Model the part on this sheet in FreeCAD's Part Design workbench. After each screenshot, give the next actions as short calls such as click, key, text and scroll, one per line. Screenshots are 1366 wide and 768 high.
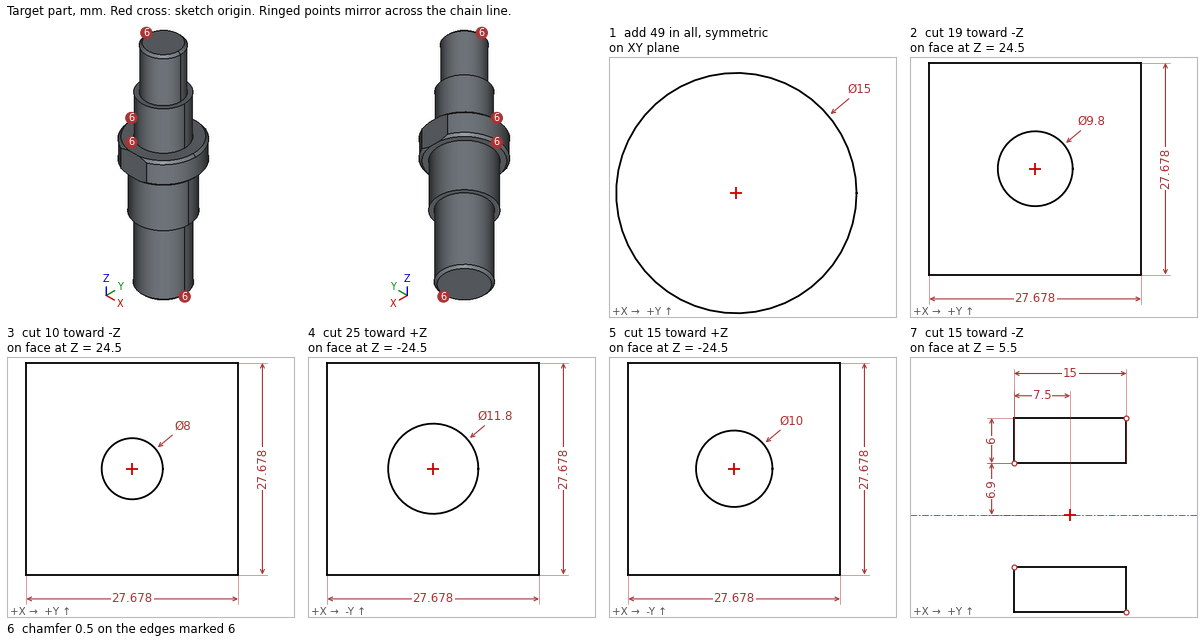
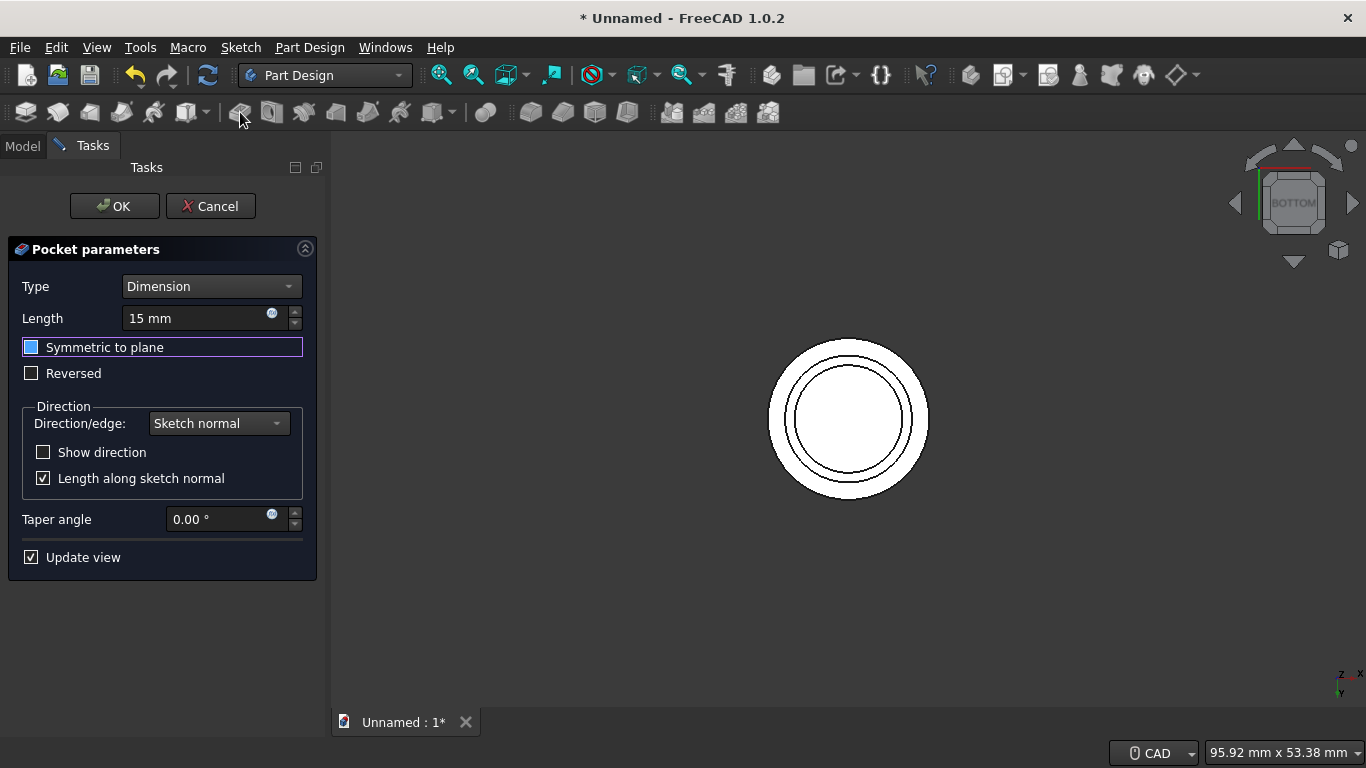
click(115, 206)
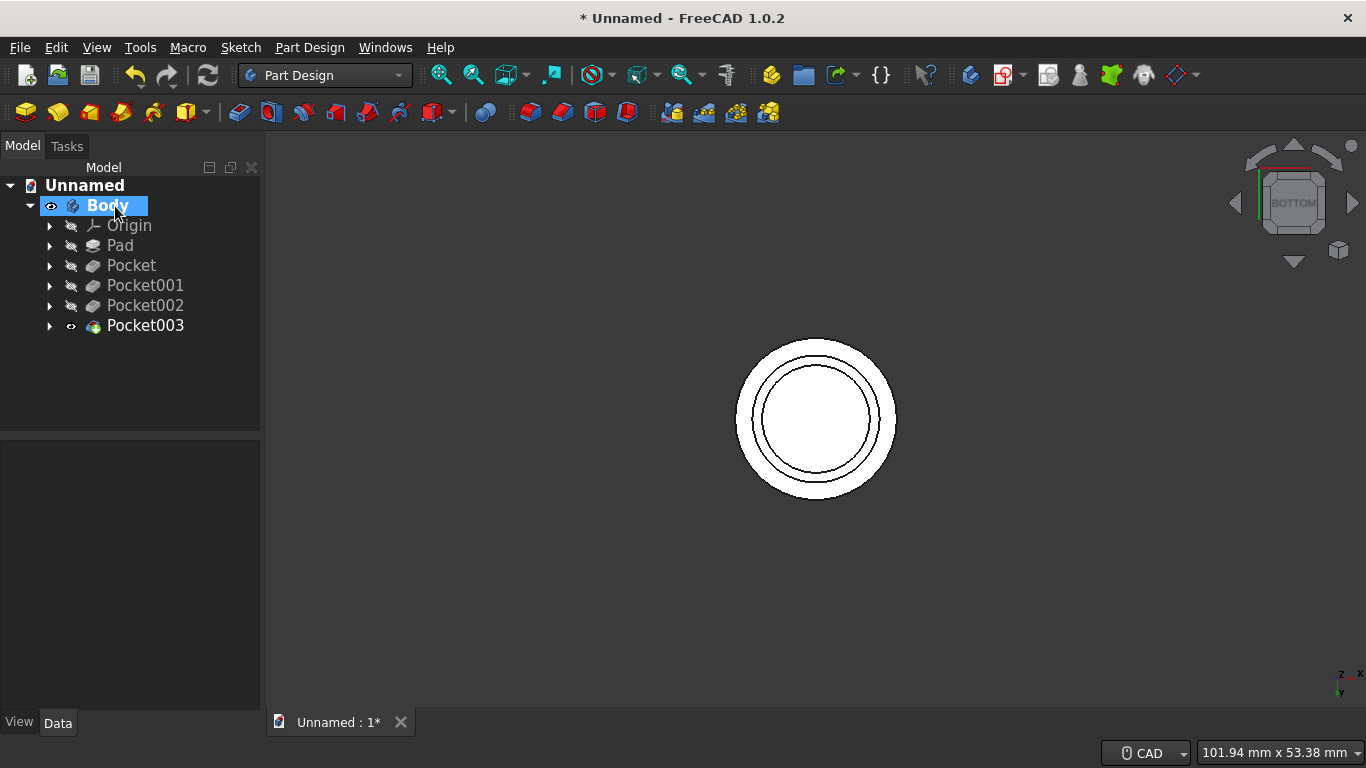
click(442, 76)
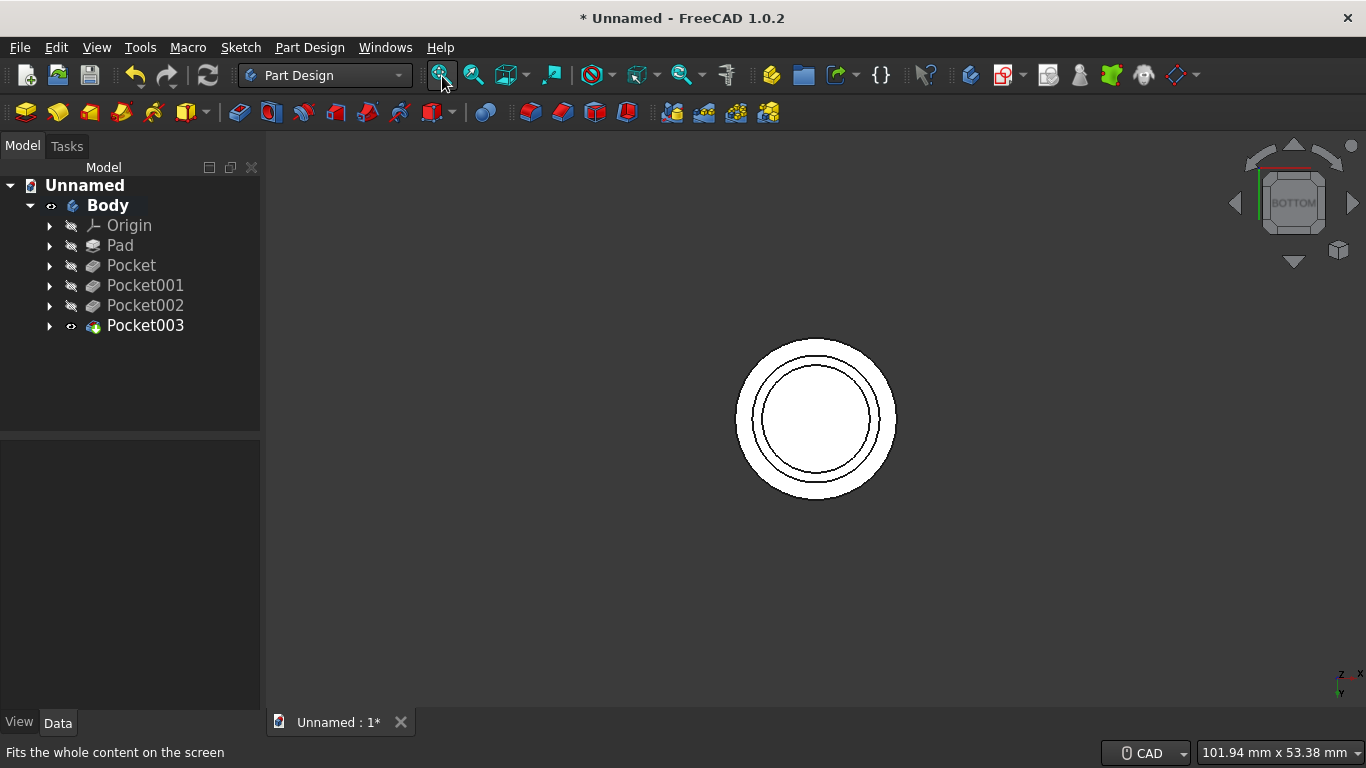
click(735, 418)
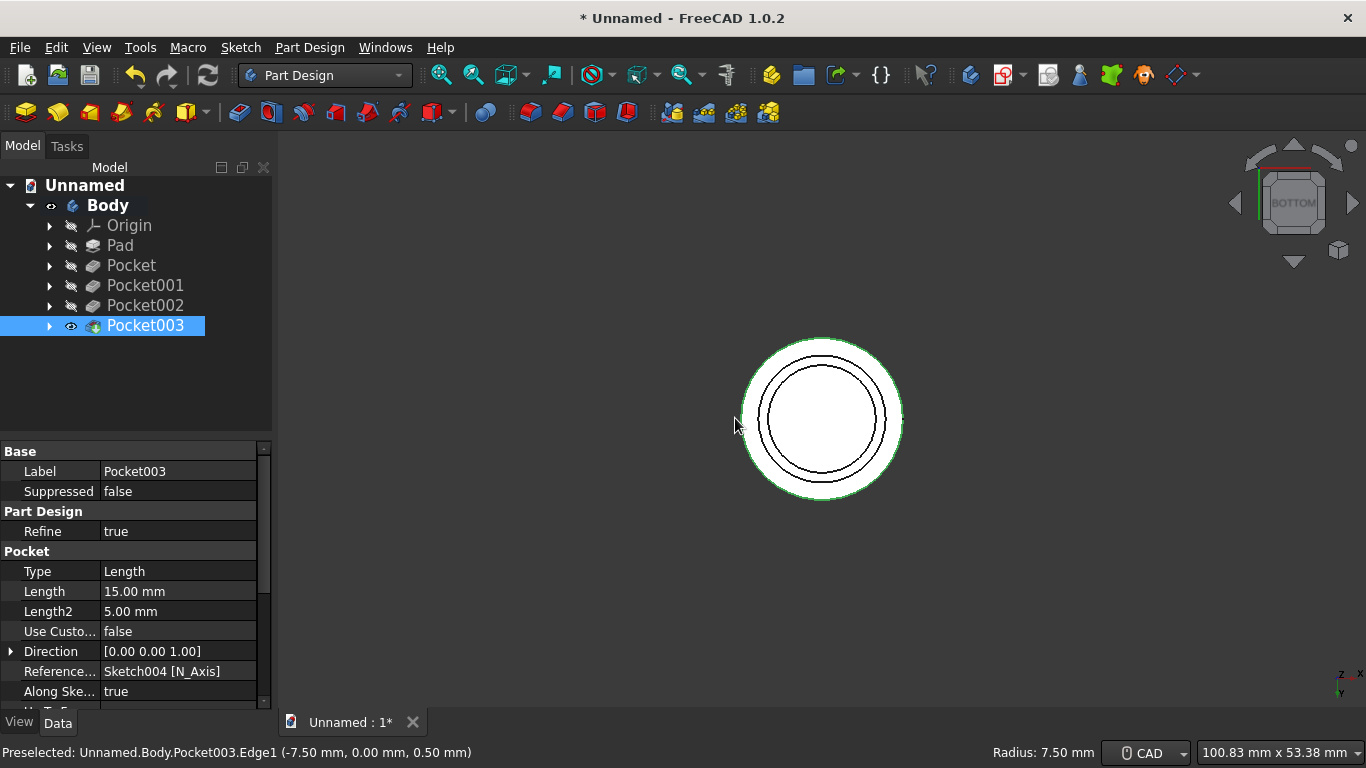
click(768, 418, ctrl)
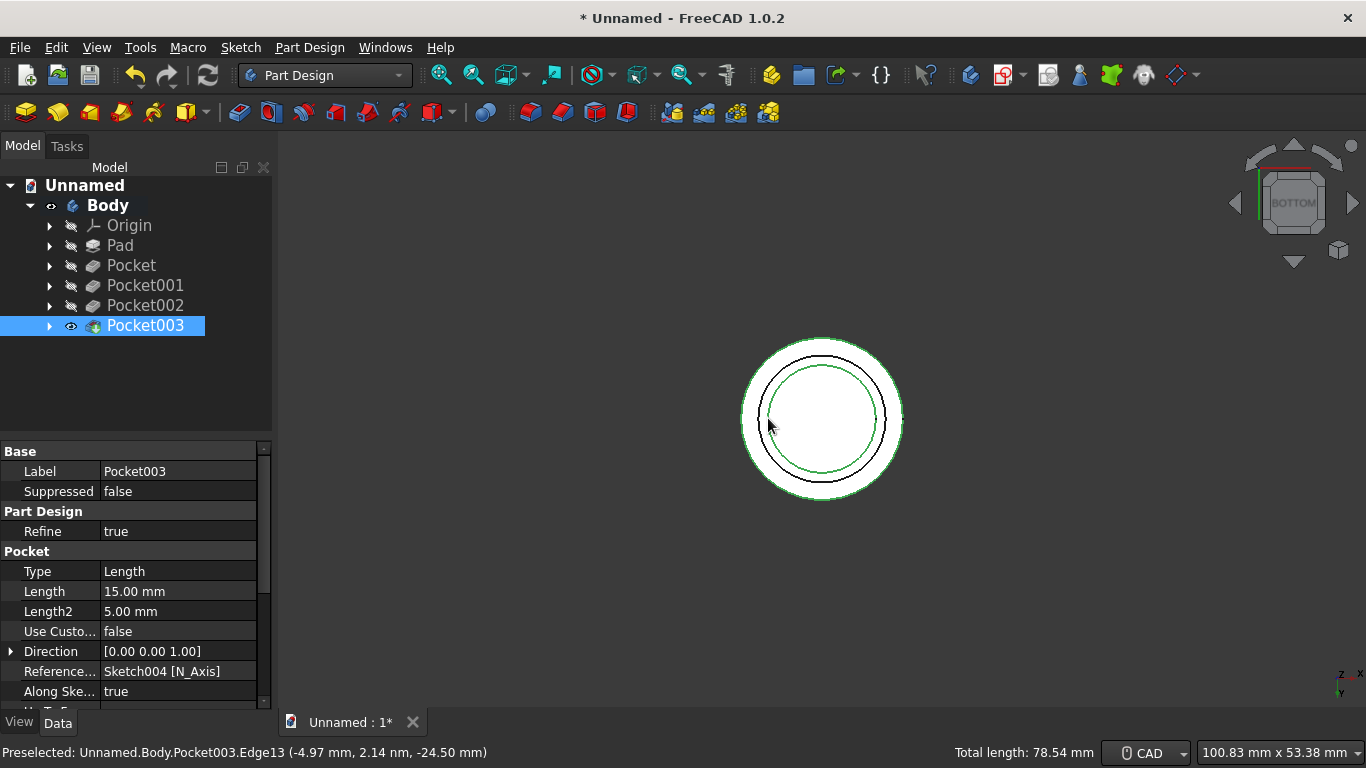
key(0)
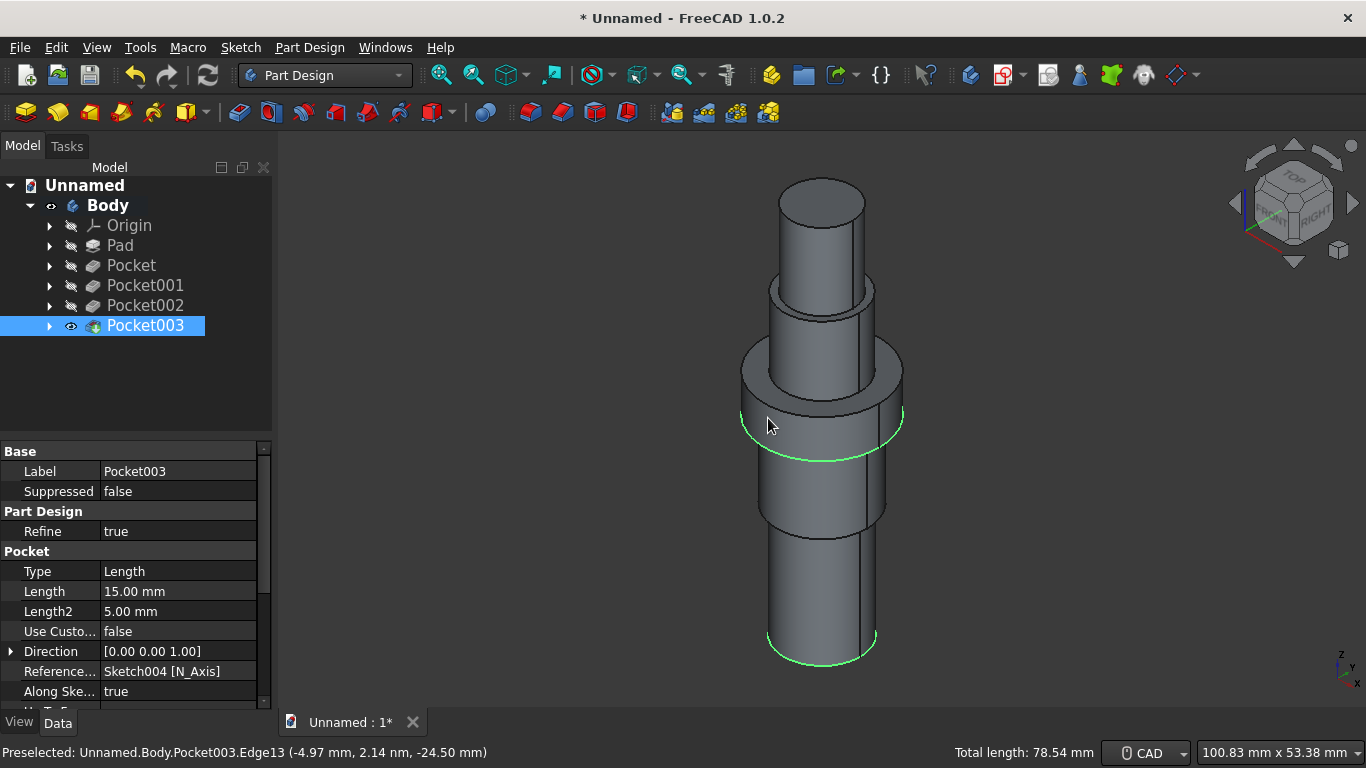
click(779, 198, ctrl)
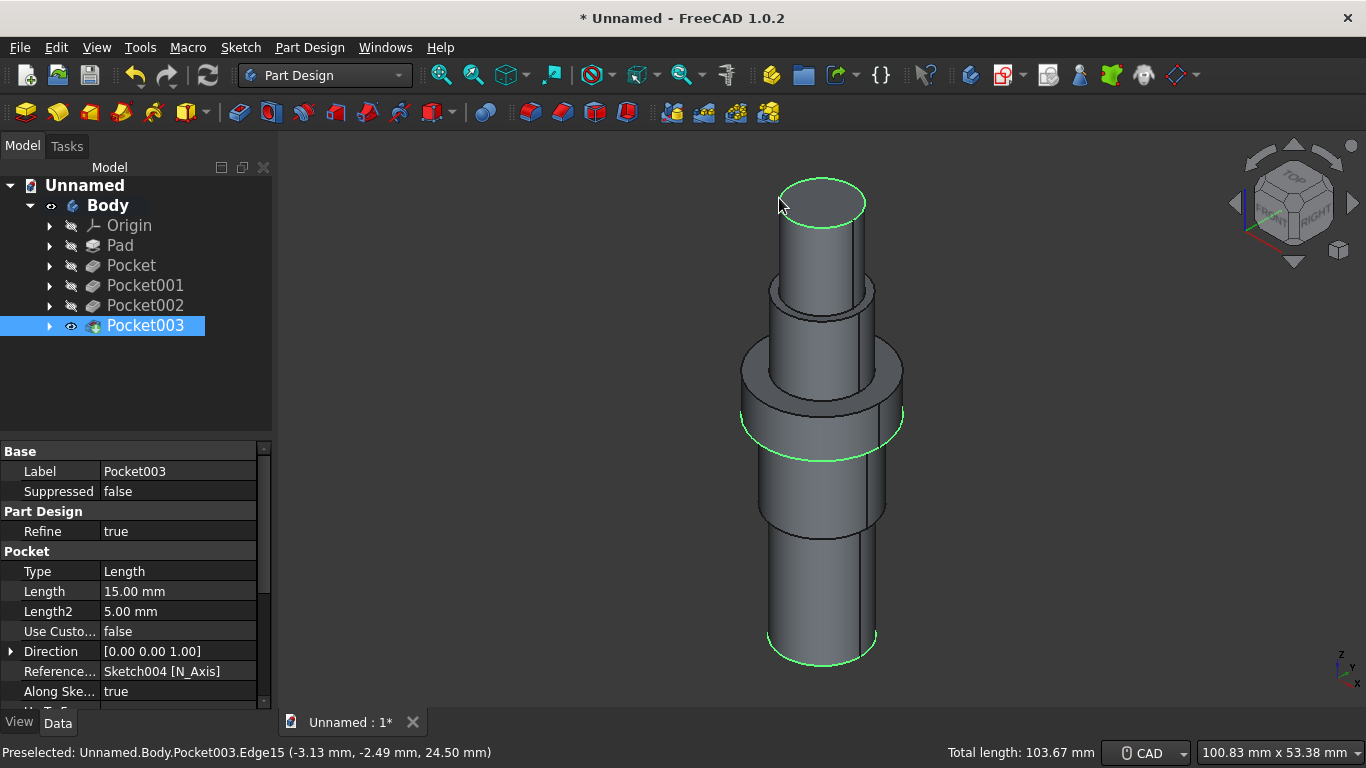
click(750, 391, ctrl)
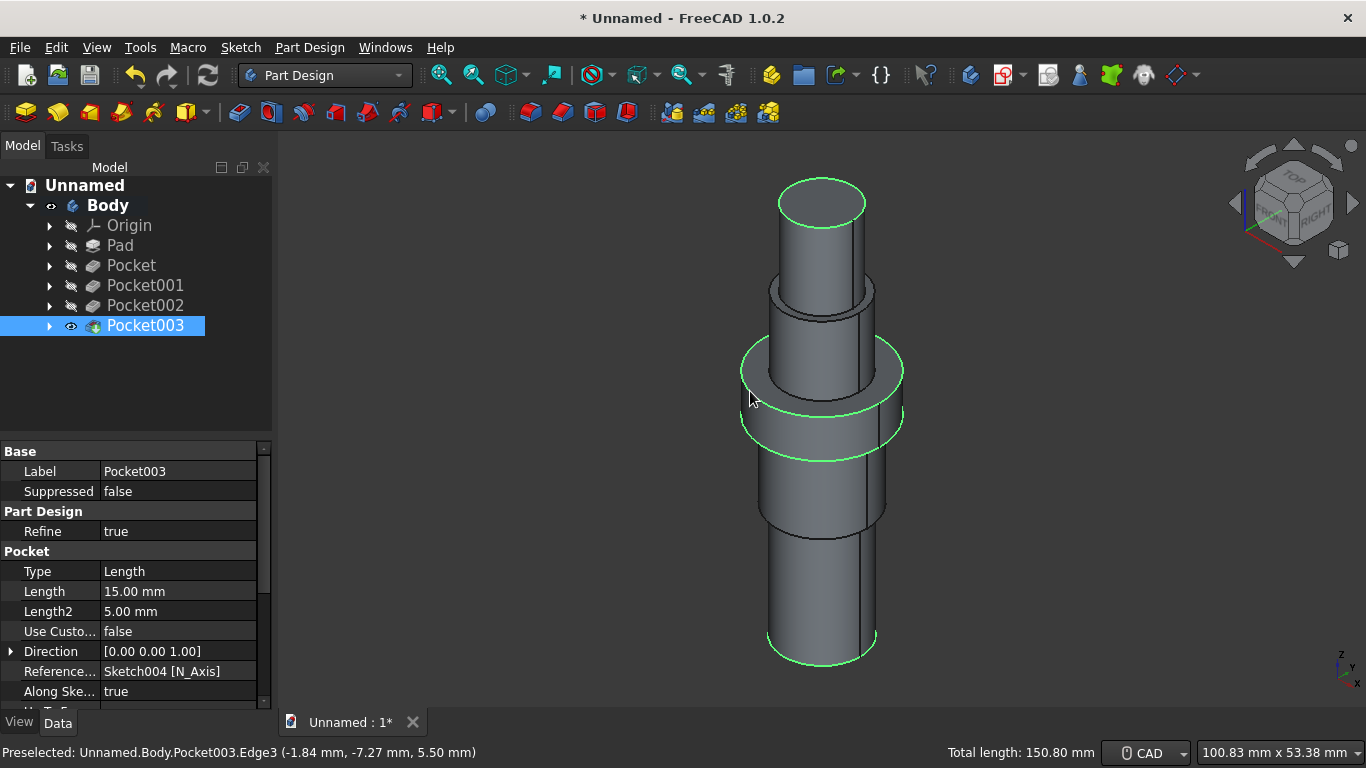
click(564, 112)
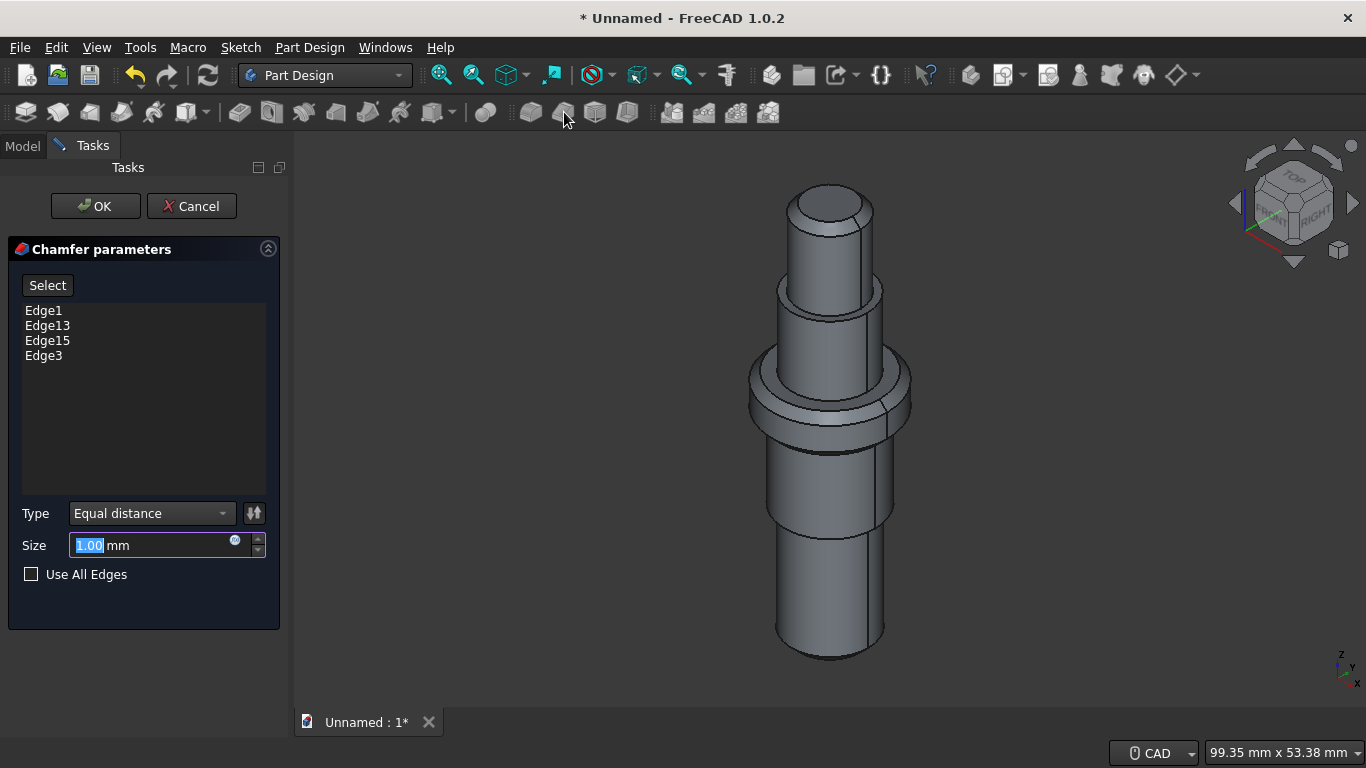
text(0.5)
key(Tab)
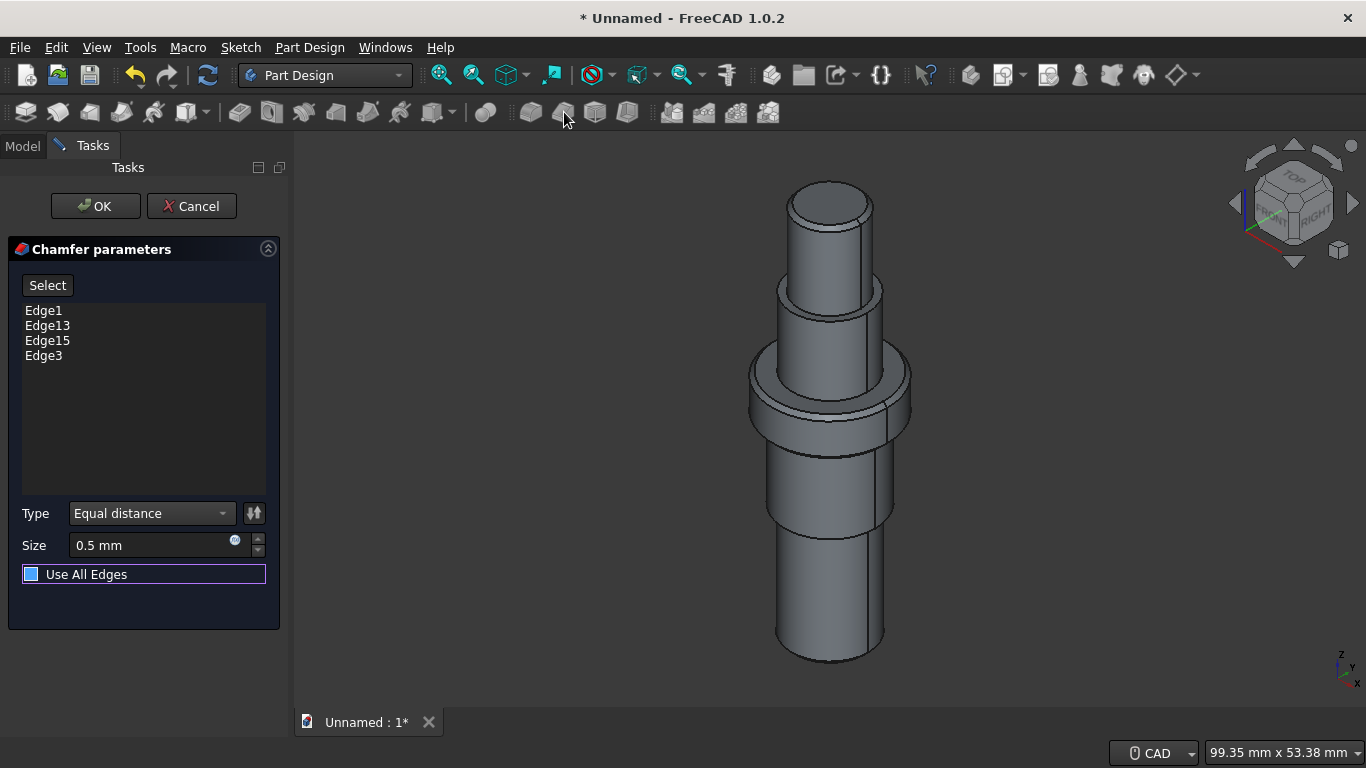
click(96, 206)